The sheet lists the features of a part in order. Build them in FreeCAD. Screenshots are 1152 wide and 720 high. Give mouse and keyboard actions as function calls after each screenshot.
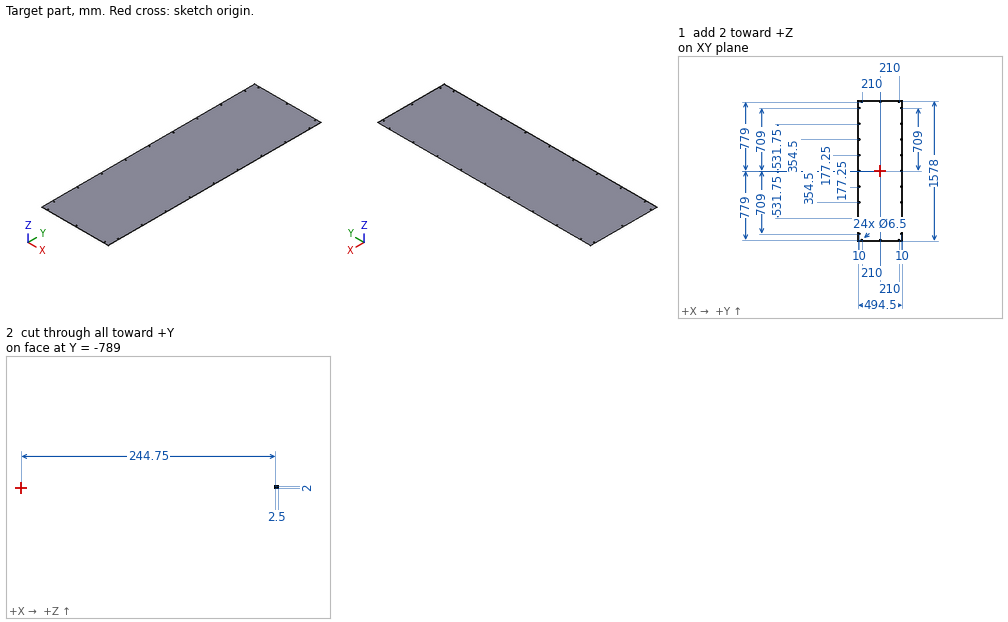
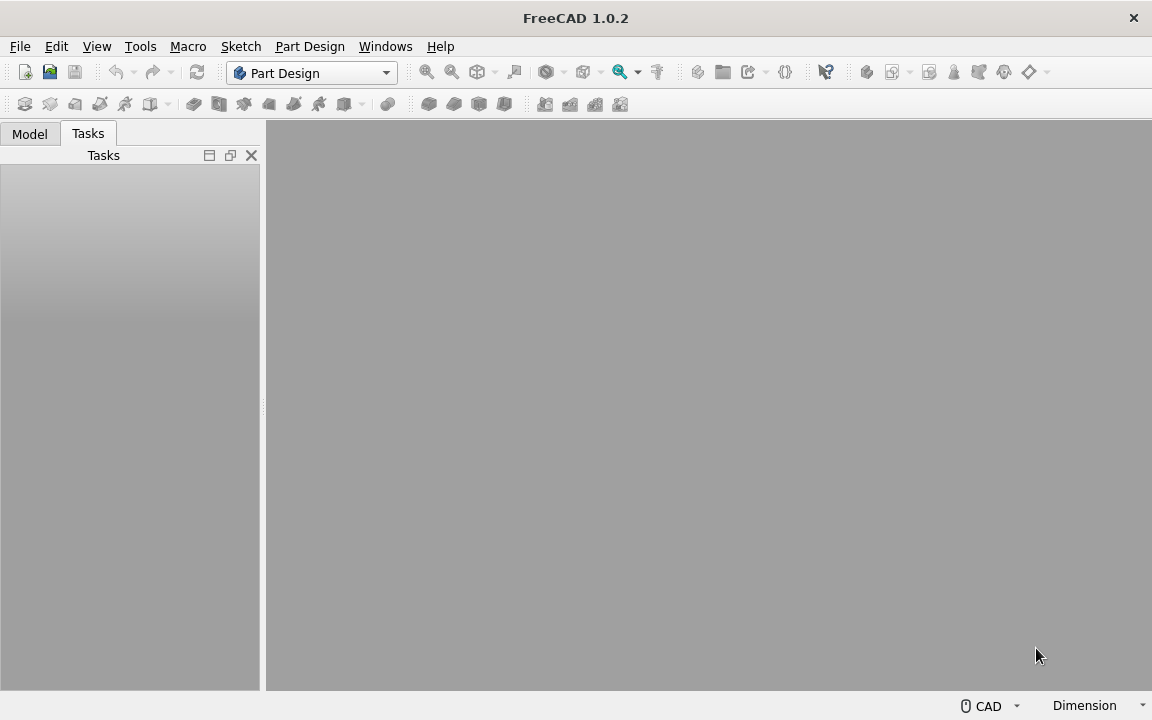
click(25, 72)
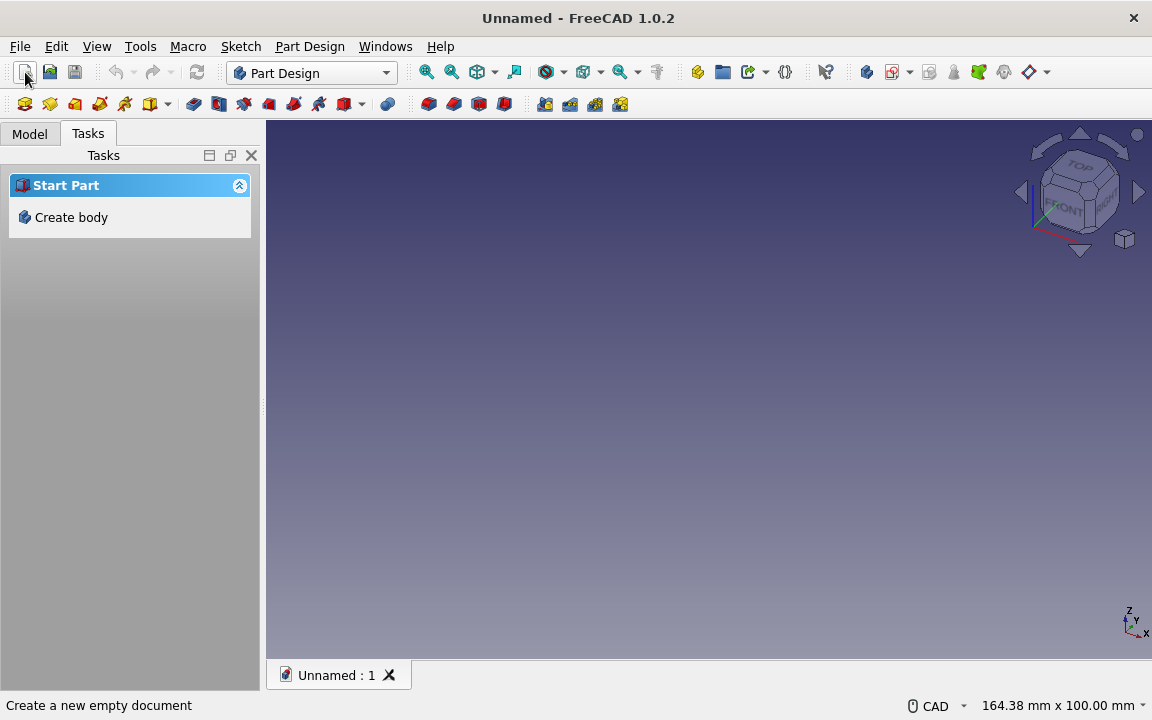
click(892, 72)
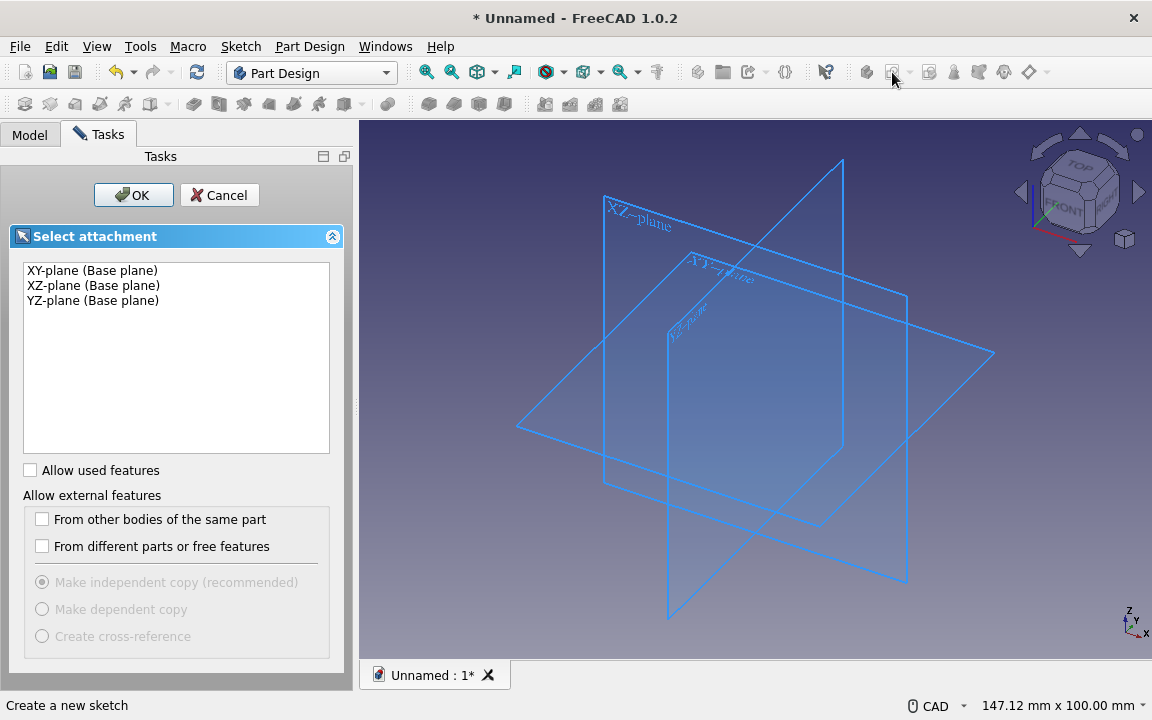
click(84, 270)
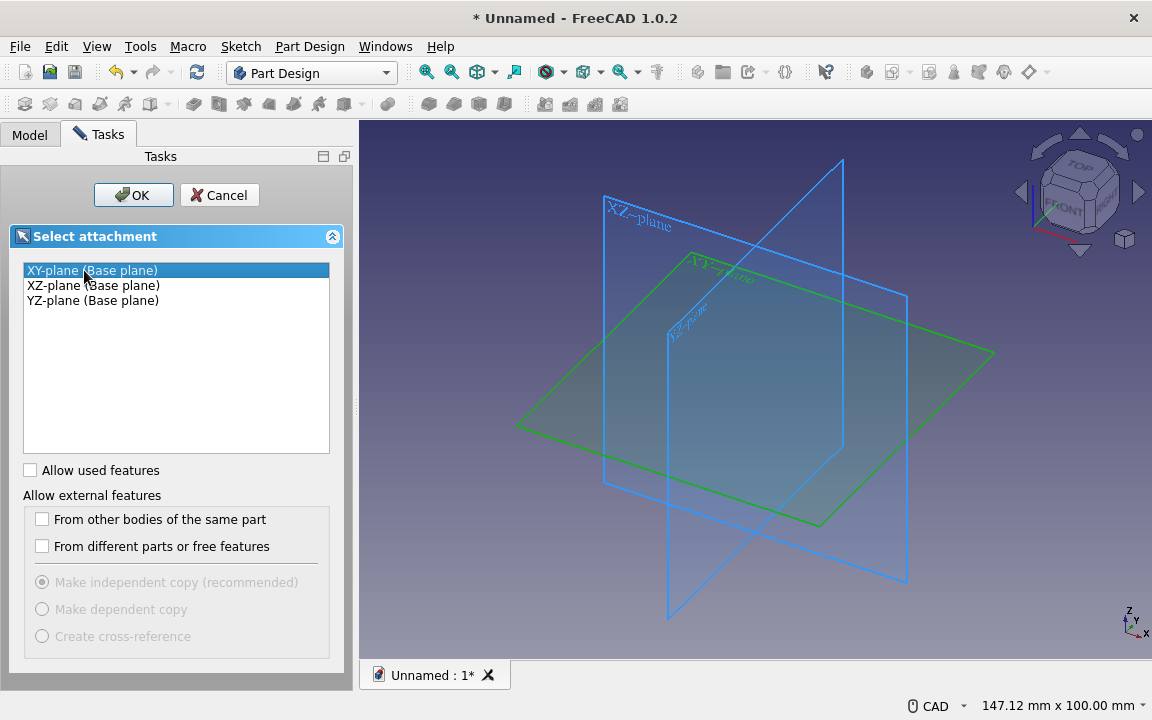
click(134, 195)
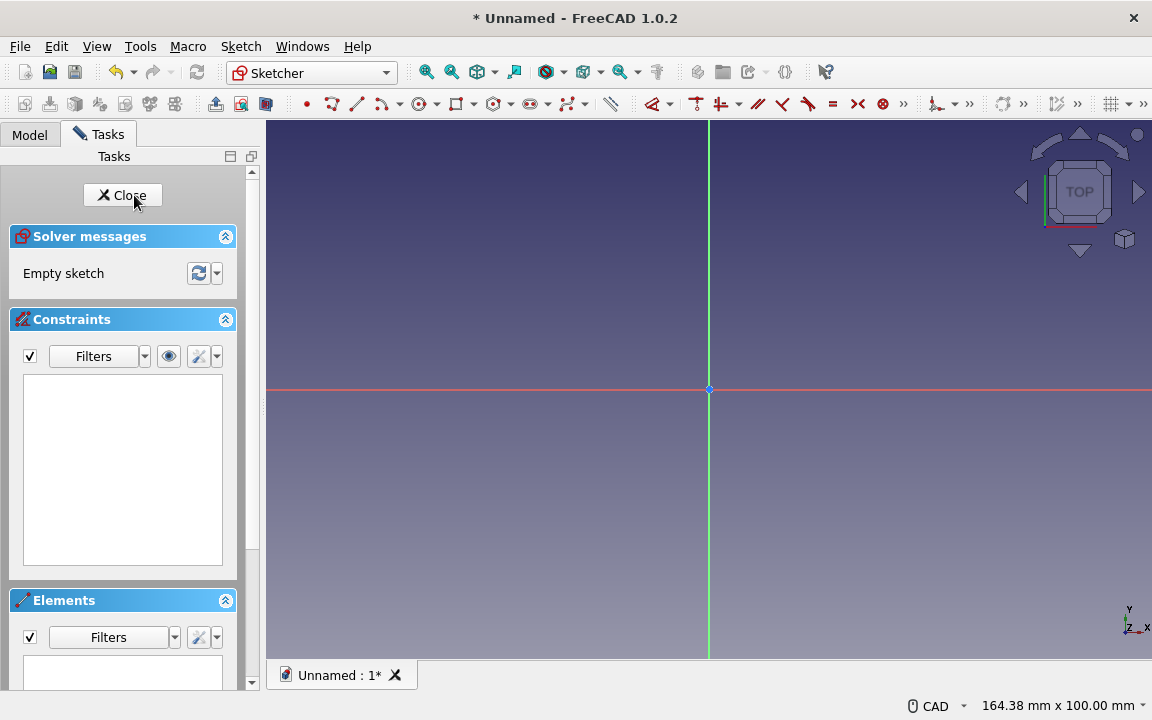
scroll(637, 390, down, 15)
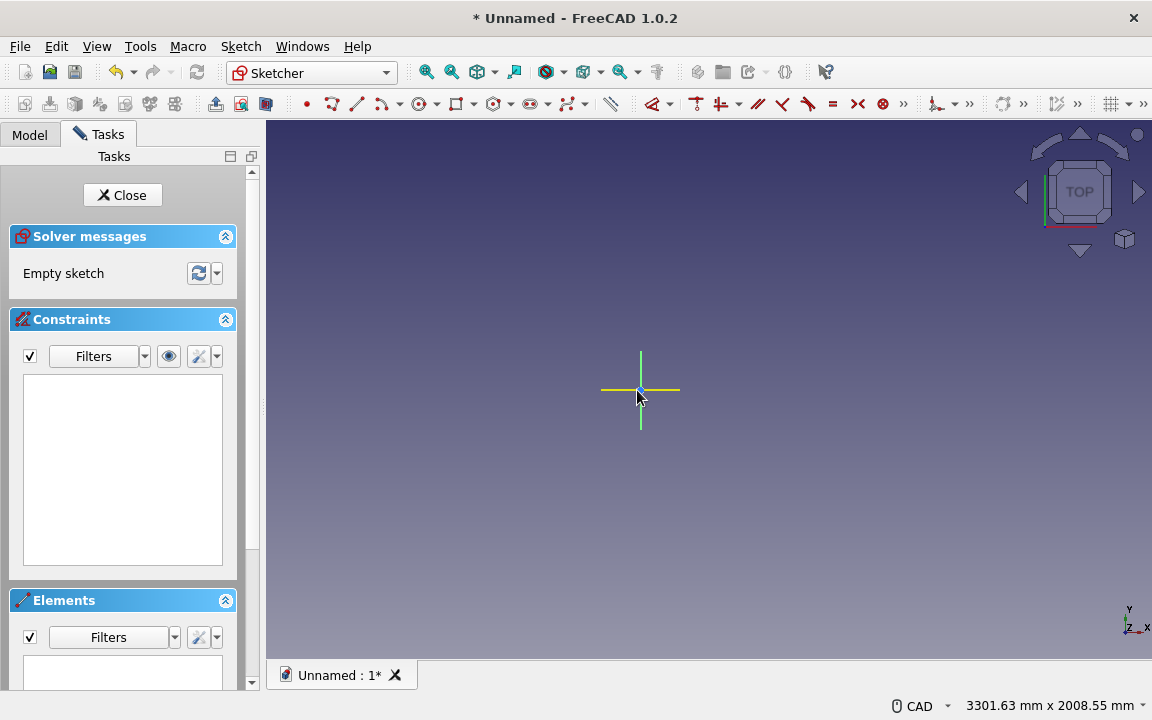
key(g)
key(v)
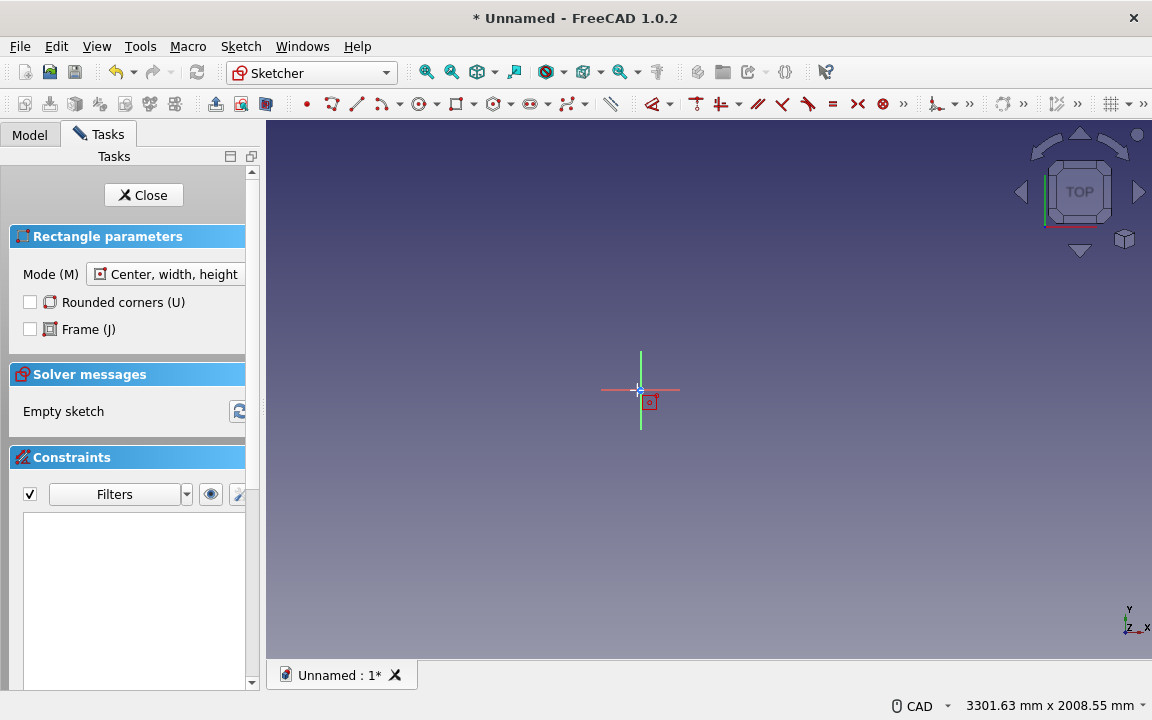
click(641, 390)
move(707, 179)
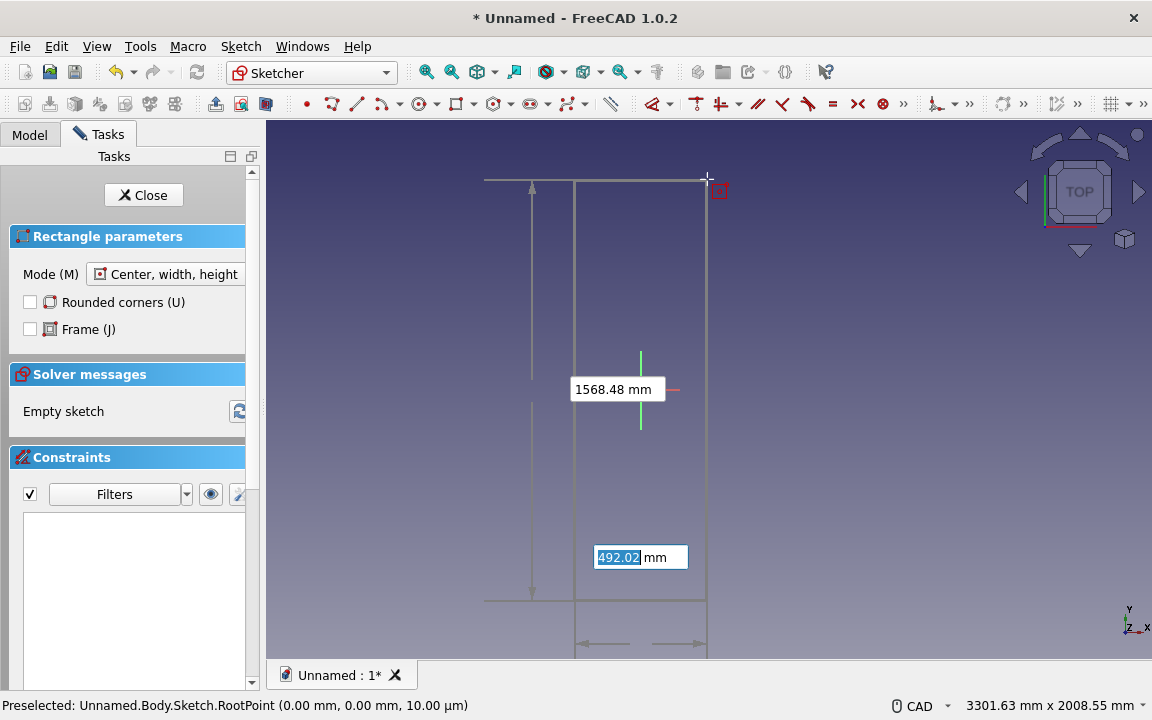
text(494.5)
key(Tab)
text(1578)
key(Return)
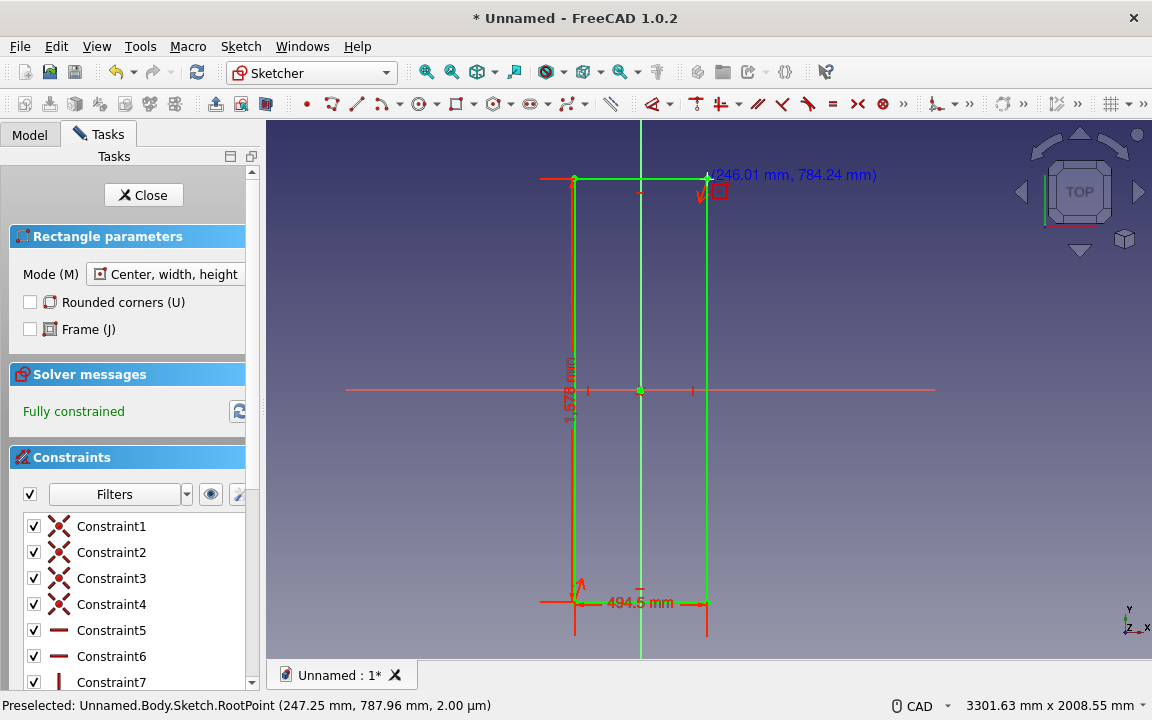
click(418, 104)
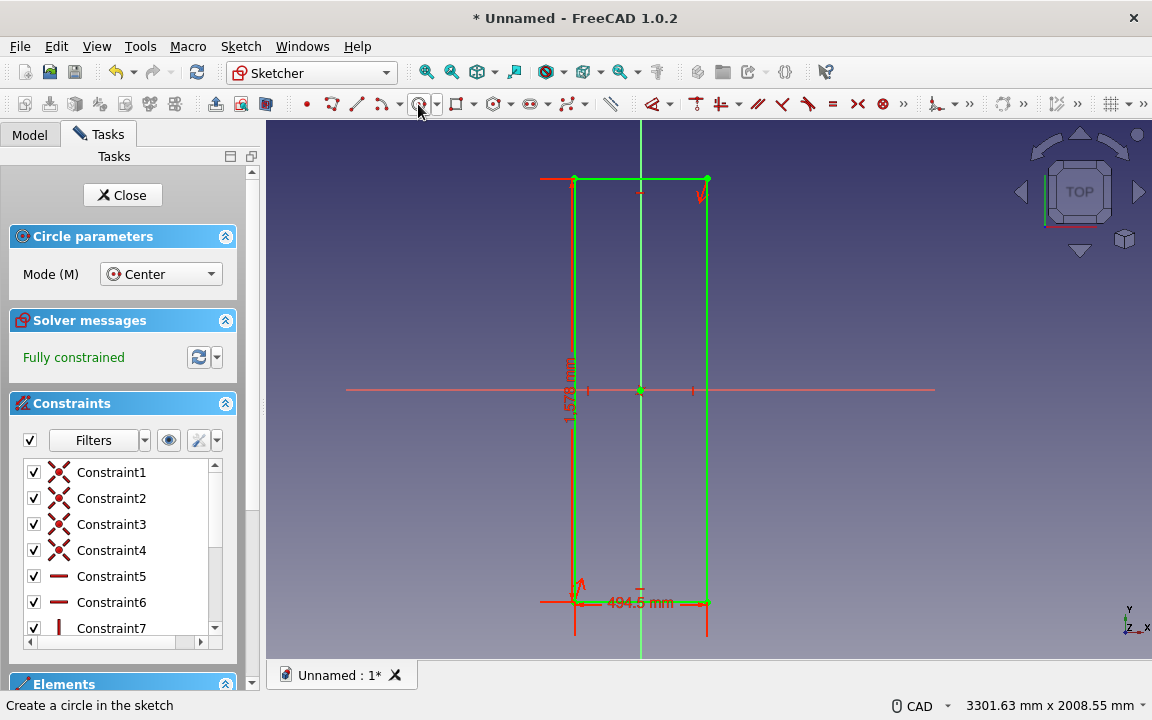
scroll(577, 581, up, 17)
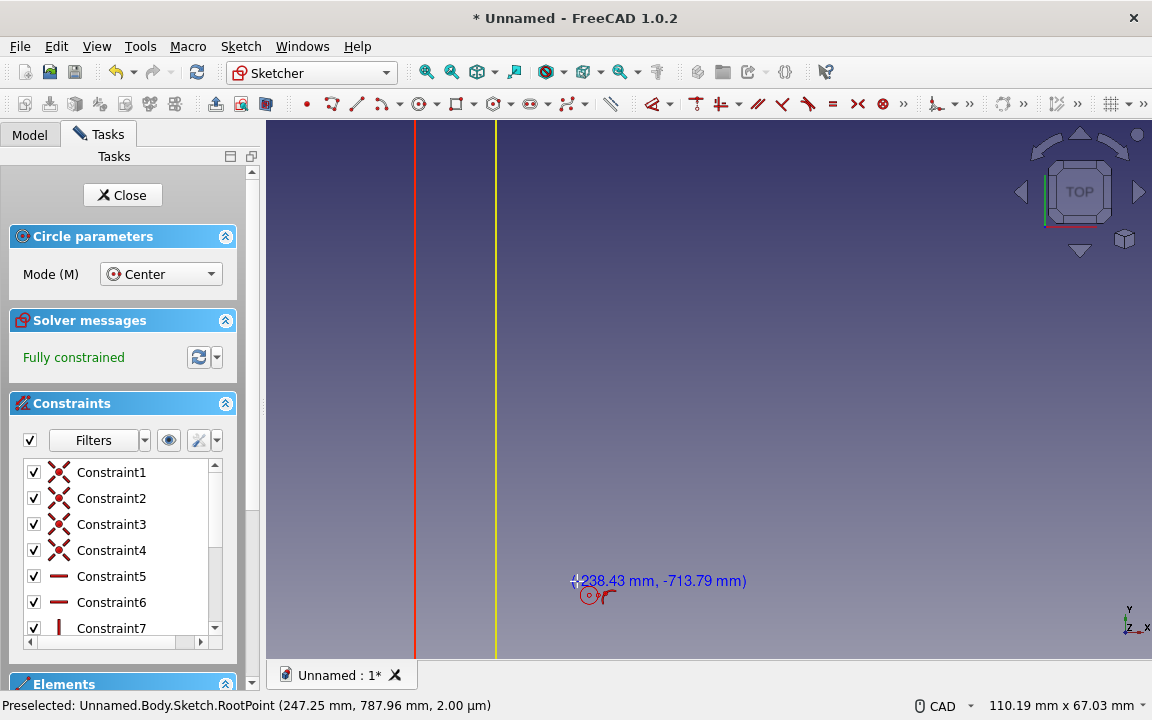
scroll(577, 581, down, 17)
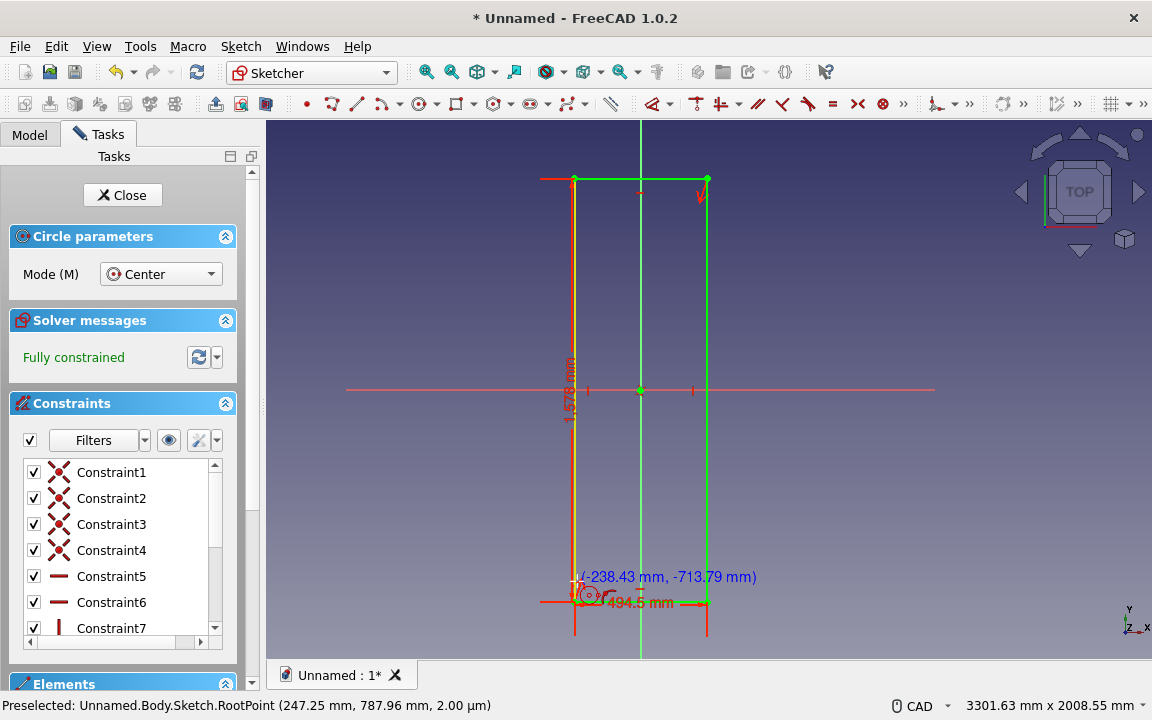
scroll(577, 581, up, 9)